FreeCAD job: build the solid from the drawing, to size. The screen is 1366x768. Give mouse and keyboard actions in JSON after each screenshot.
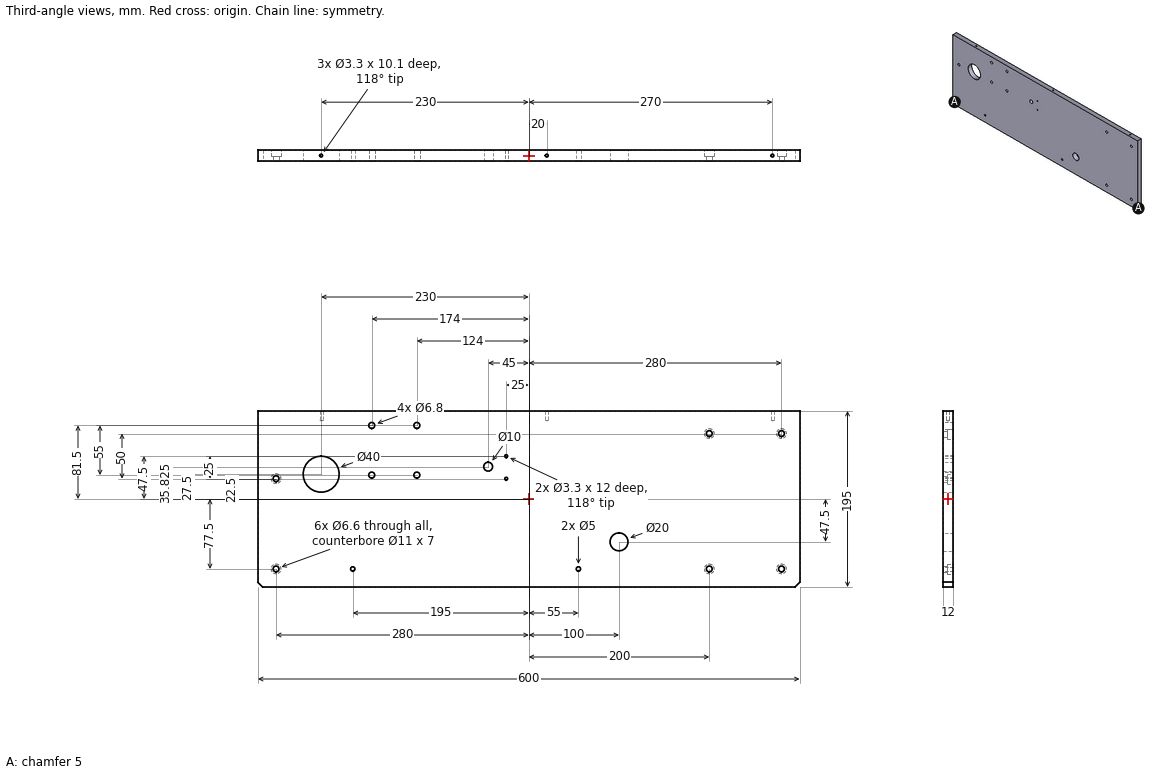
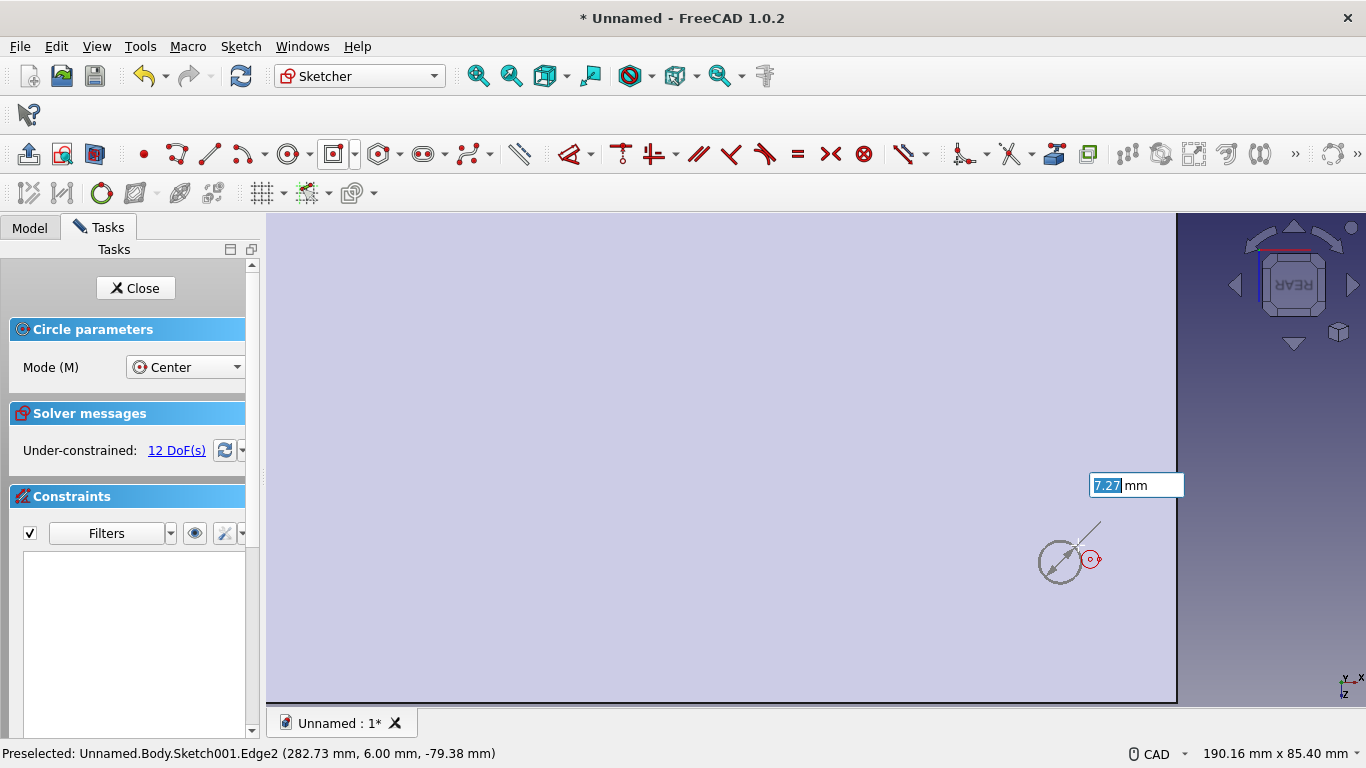
{"action": "left_click", "coordinate": [1075, 545]}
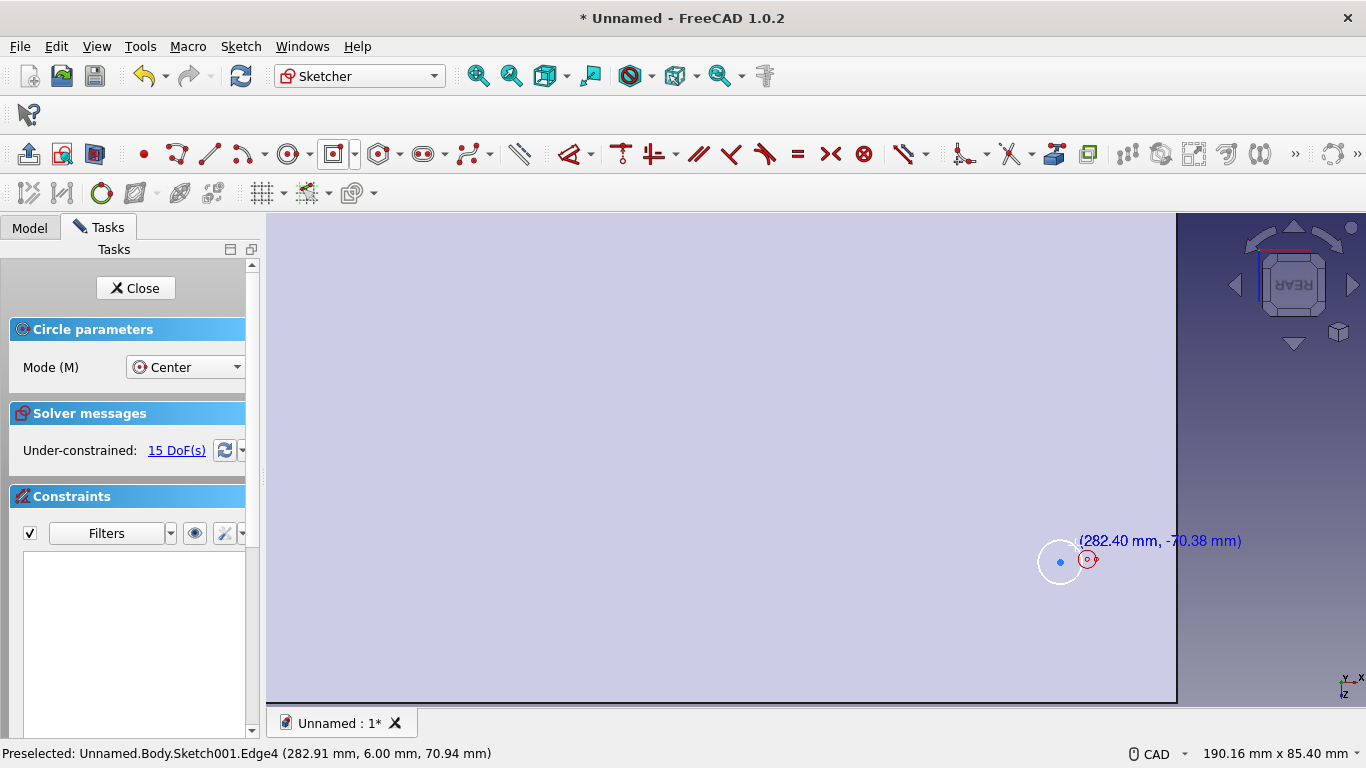
{"action": "scroll", "coordinate": [1078, 545], "scroll_direction": "down", "scroll_amount": 8}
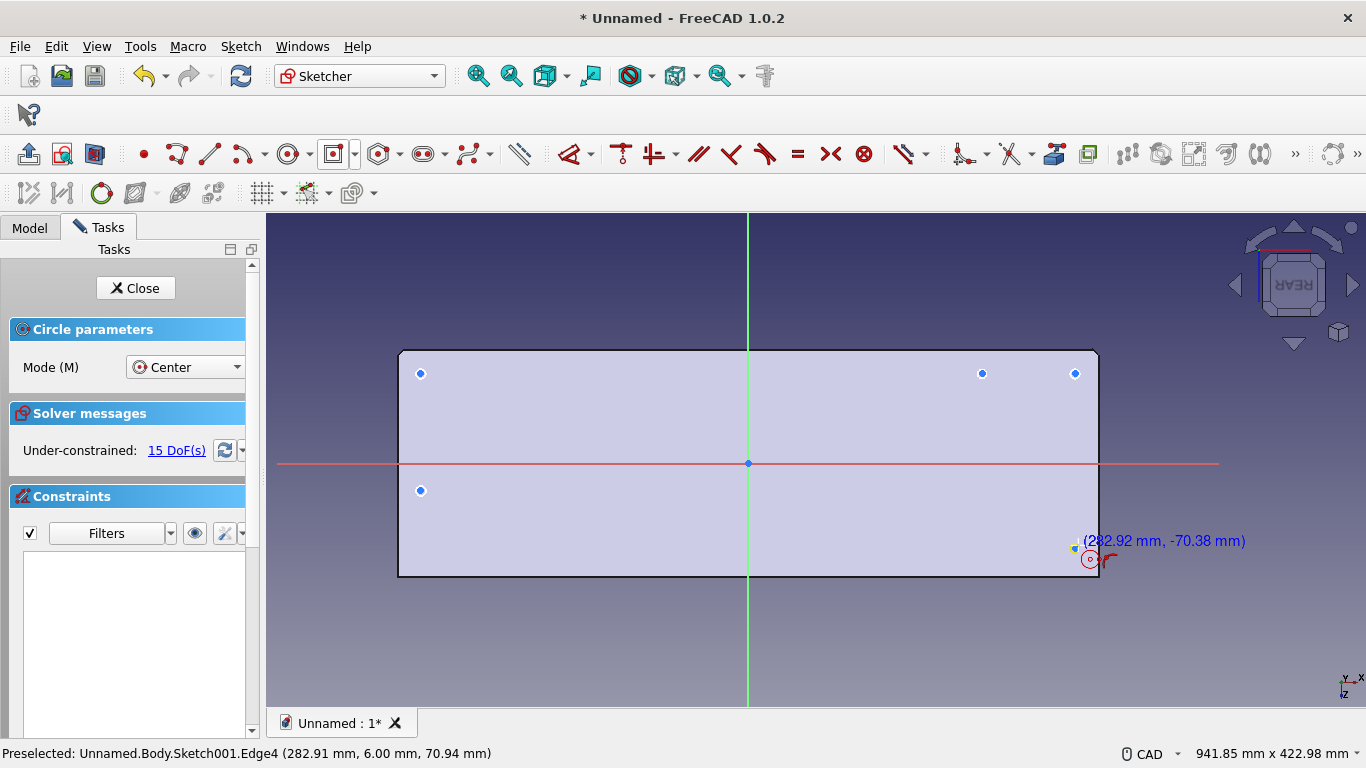
{"action": "left_click", "coordinate": [982, 548]}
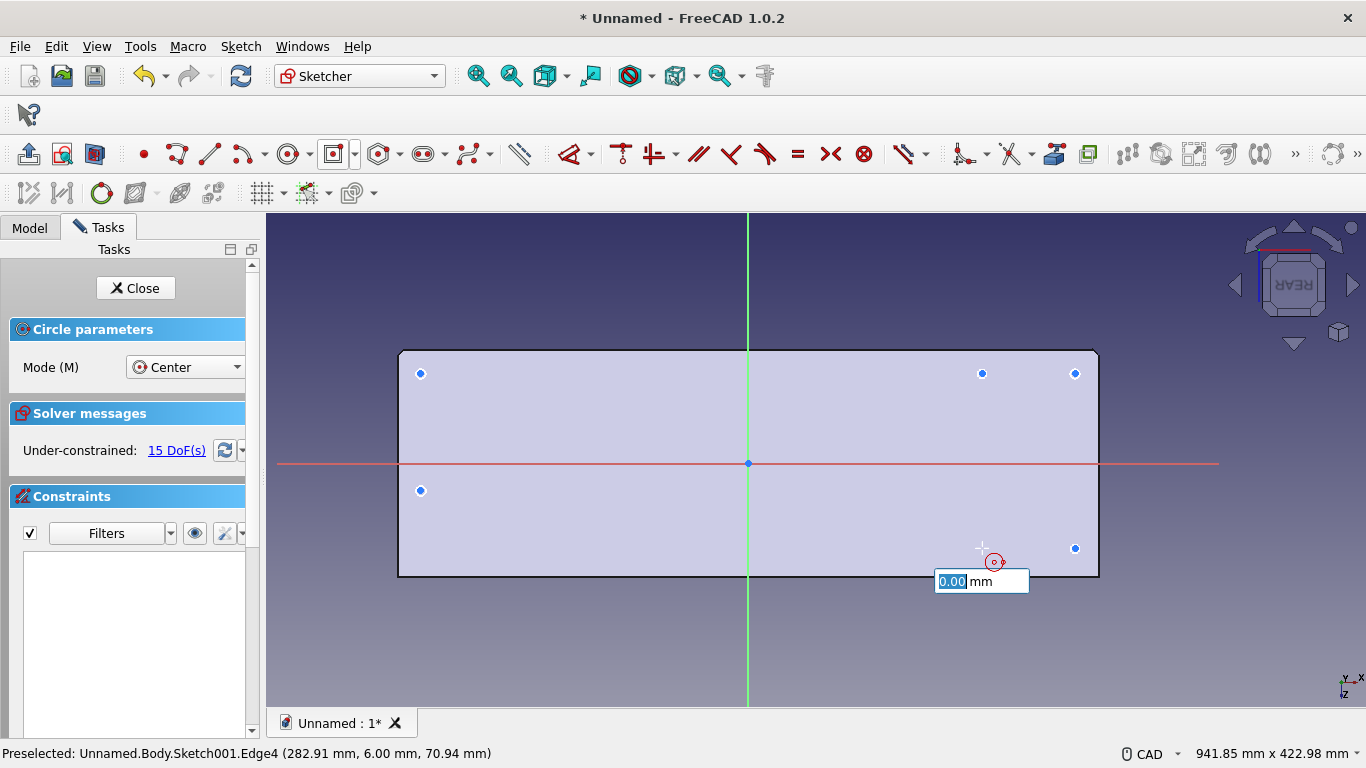
{"action": "scroll", "coordinate": [984, 545], "scroll_direction": "up", "scroll_amount": 8}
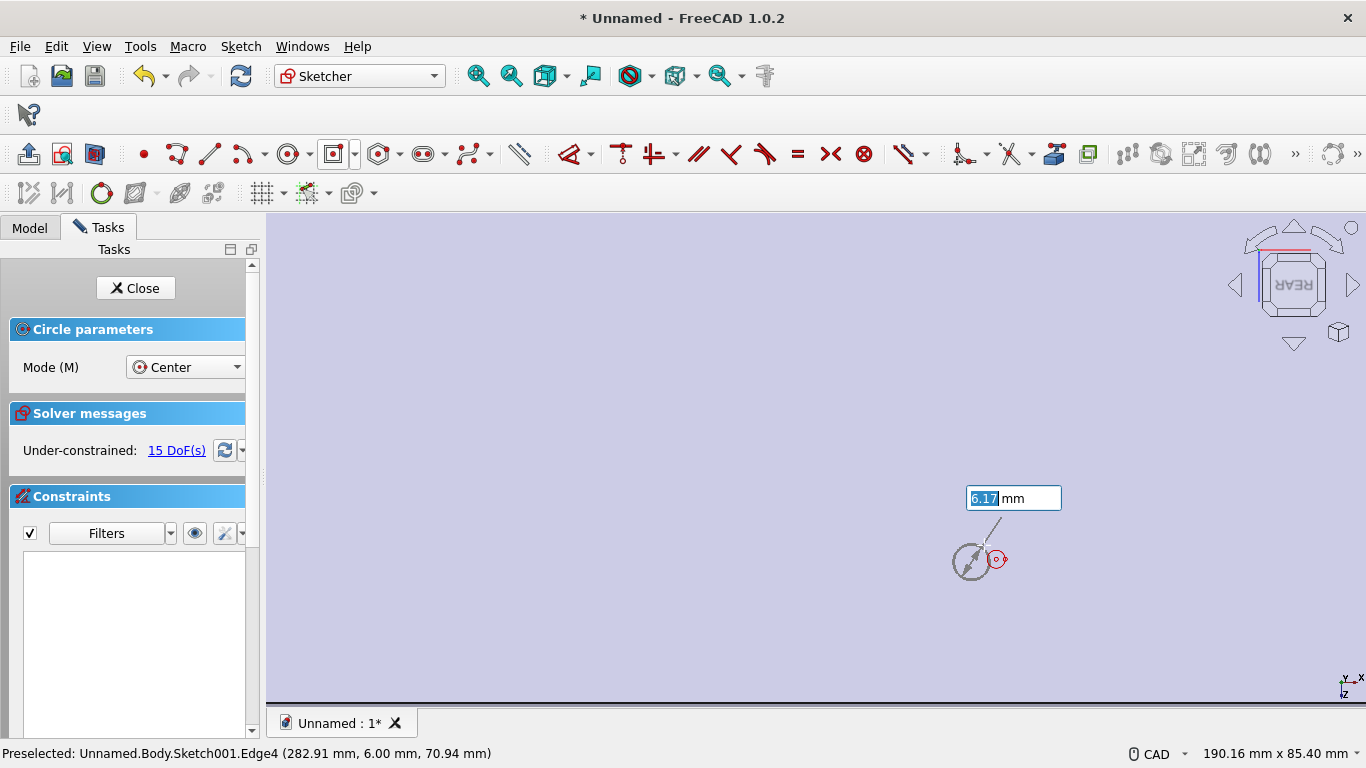
{"action": "left_click", "coordinate": [984, 545]}
{"action": "key", "text": "Escape"}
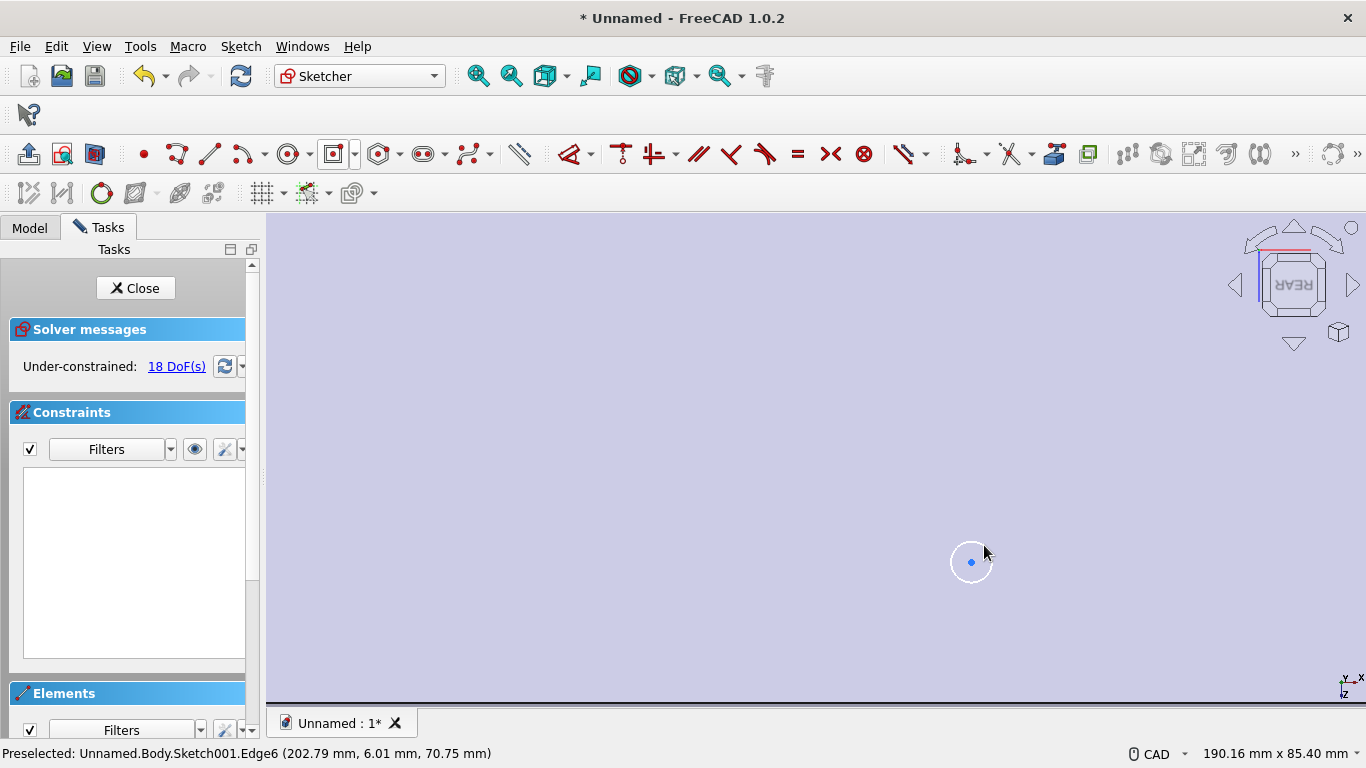
{"action": "scroll", "coordinate": [984, 545], "scroll_direction": "down", "scroll_amount": 8}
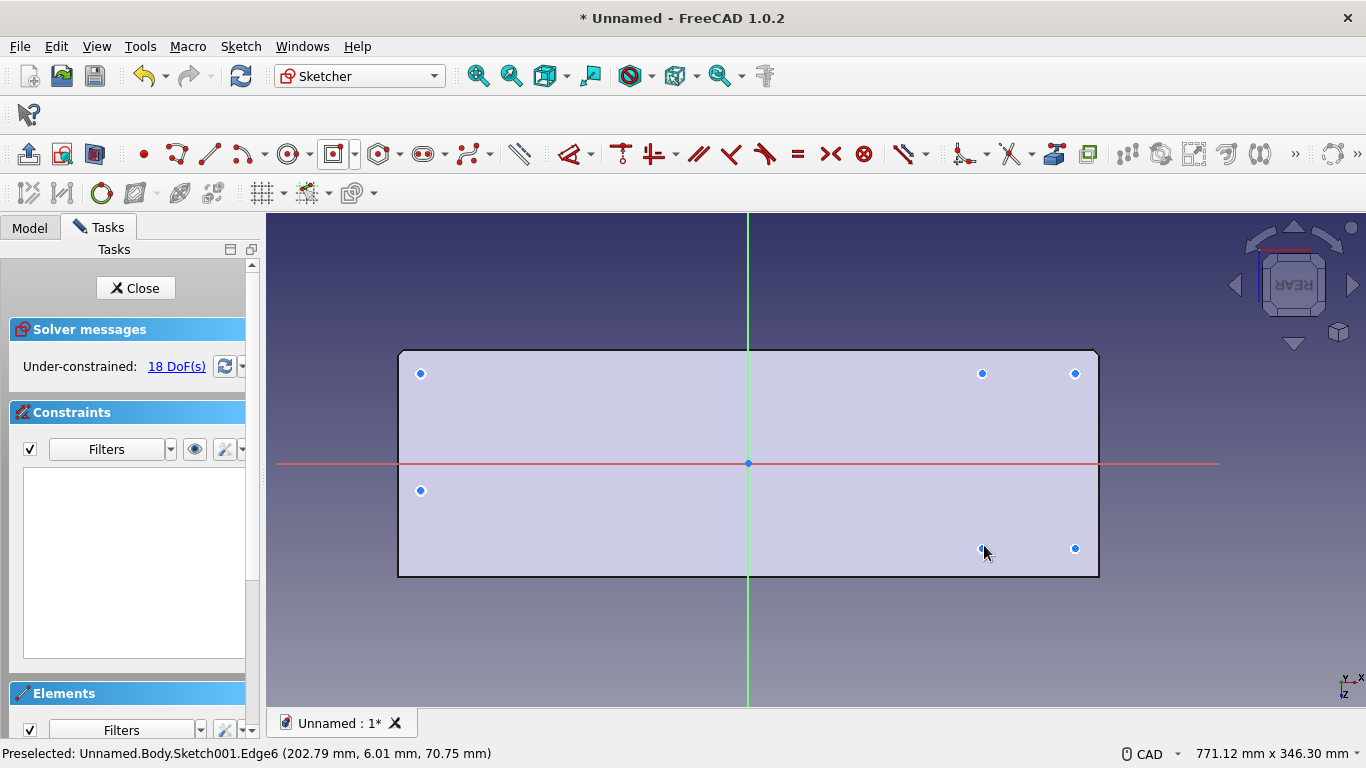
{"action": "scroll", "coordinate": [424, 371], "scroll_direction": "up", "scroll_amount": 6}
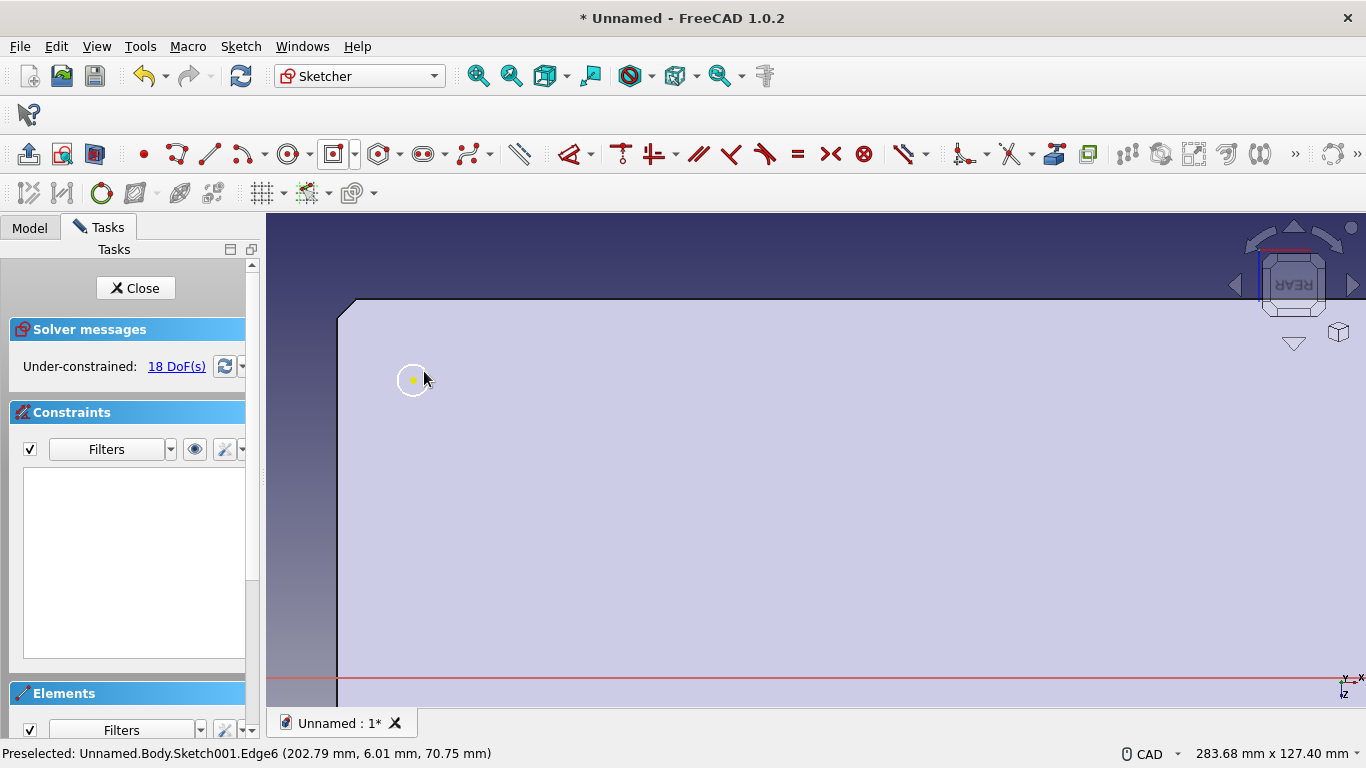
{"action": "left_click", "coordinate": [424, 369]}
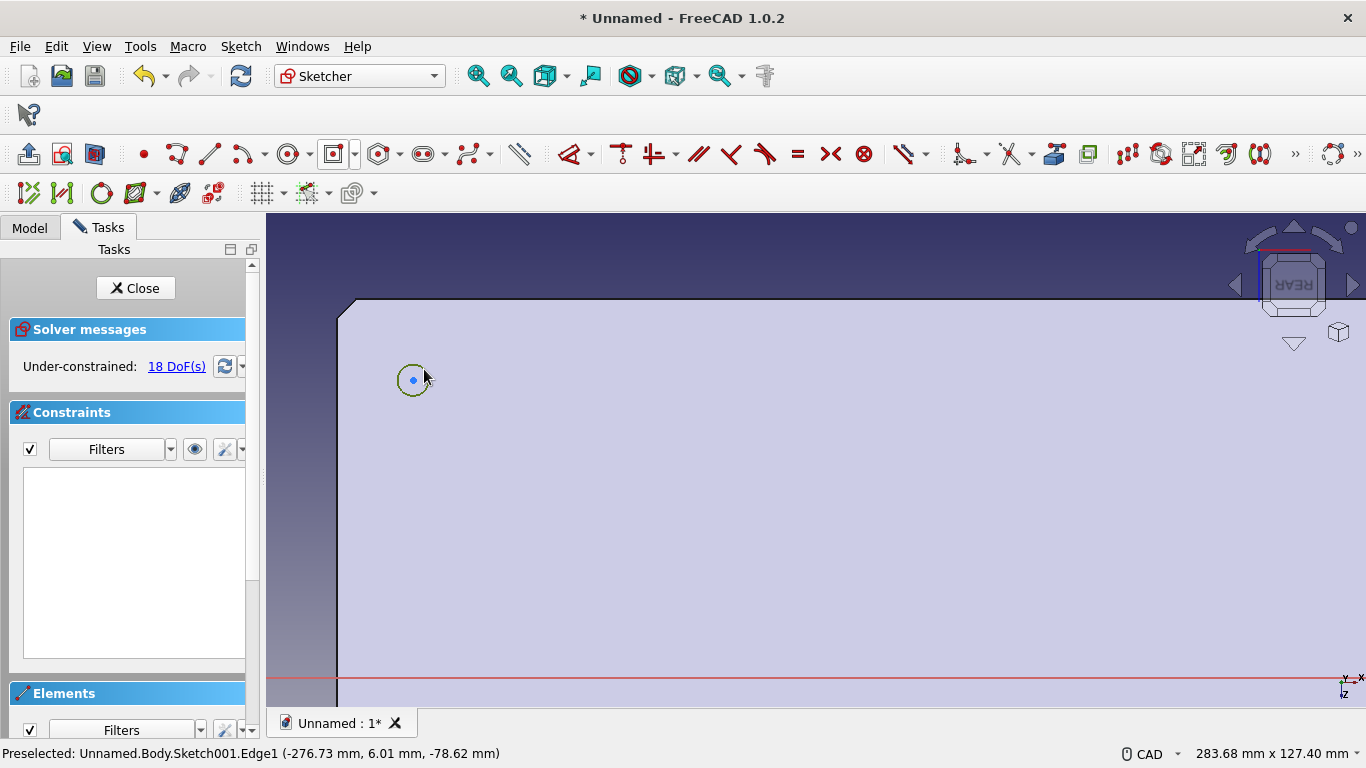
{"action": "scroll", "coordinate": [423, 370], "scroll_direction": "down", "scroll_amount": 6}